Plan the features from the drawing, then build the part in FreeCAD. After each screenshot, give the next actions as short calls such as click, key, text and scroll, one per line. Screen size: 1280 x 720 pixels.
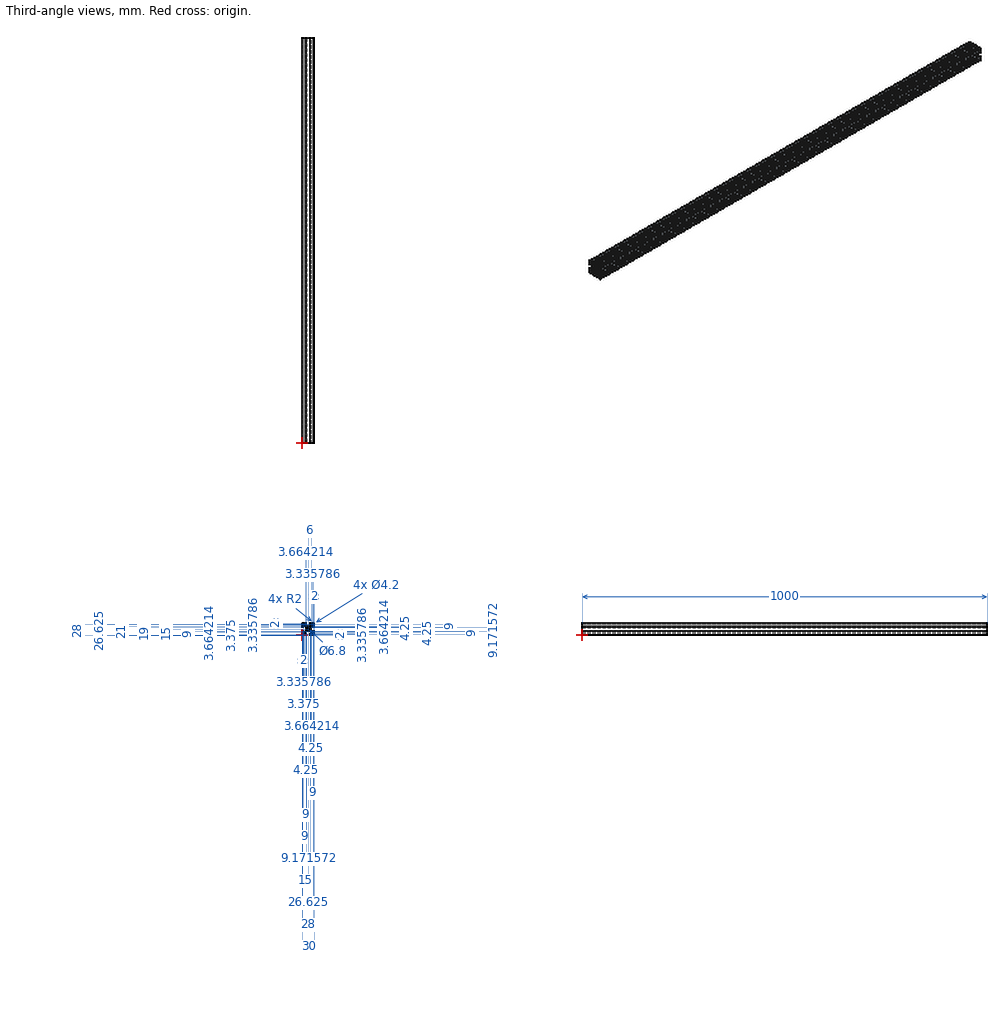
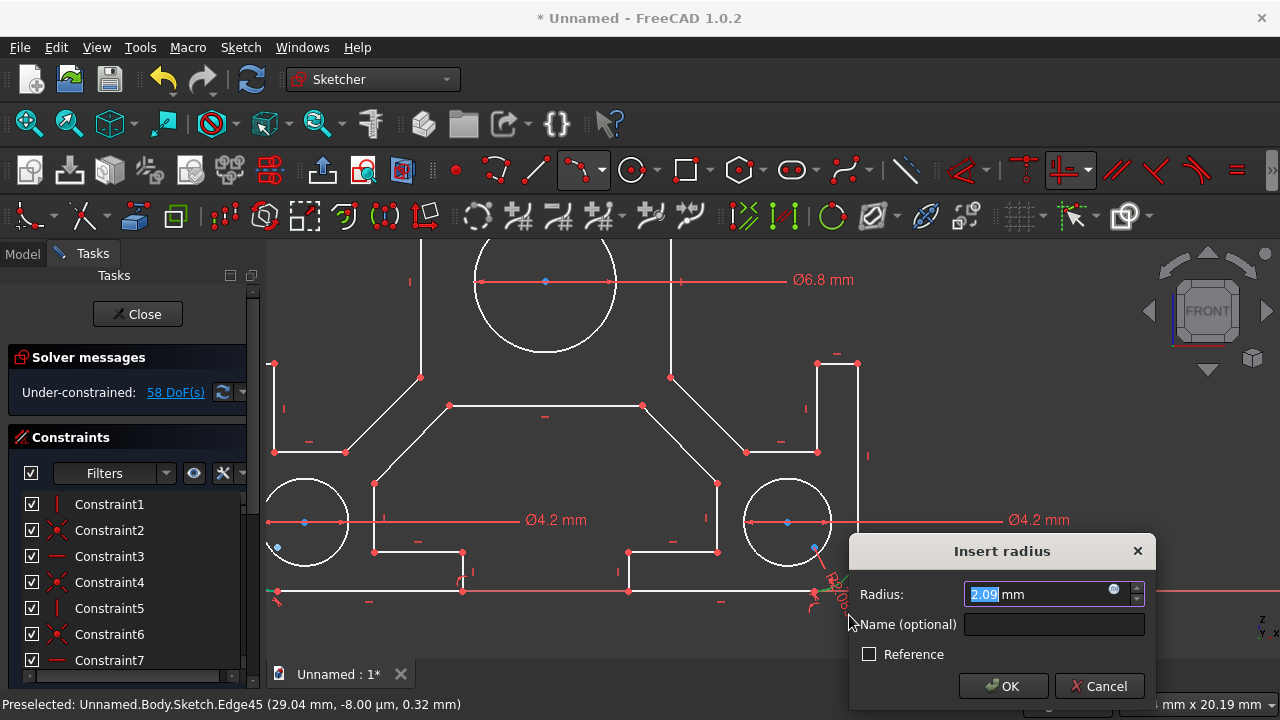
text(2)
key(Return)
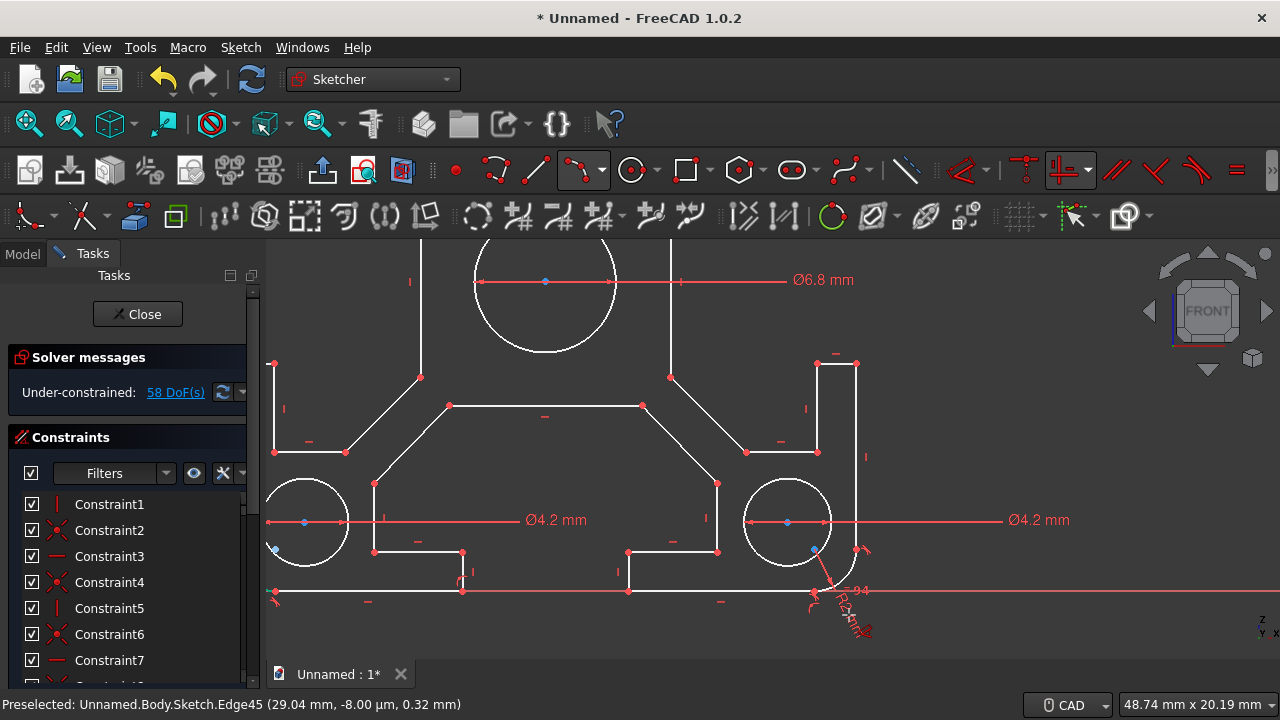
scroll(834, 588, down, 4)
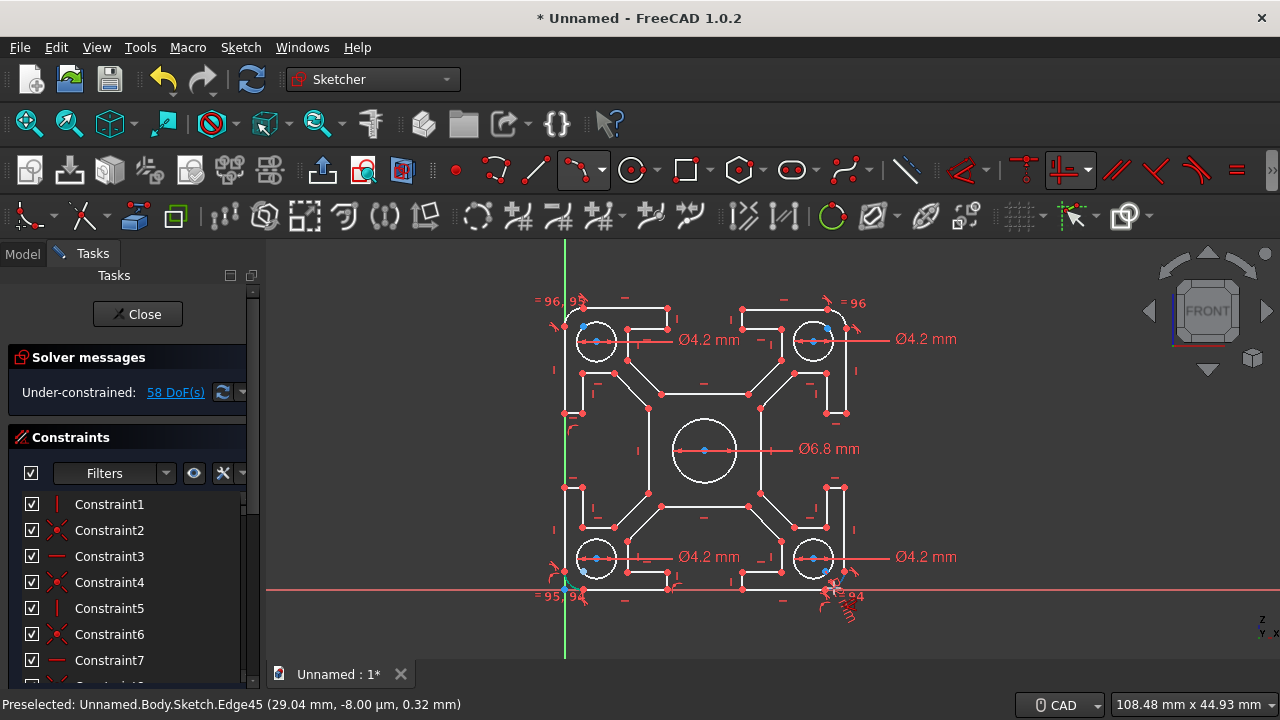
click(846, 354)
click(880, 371)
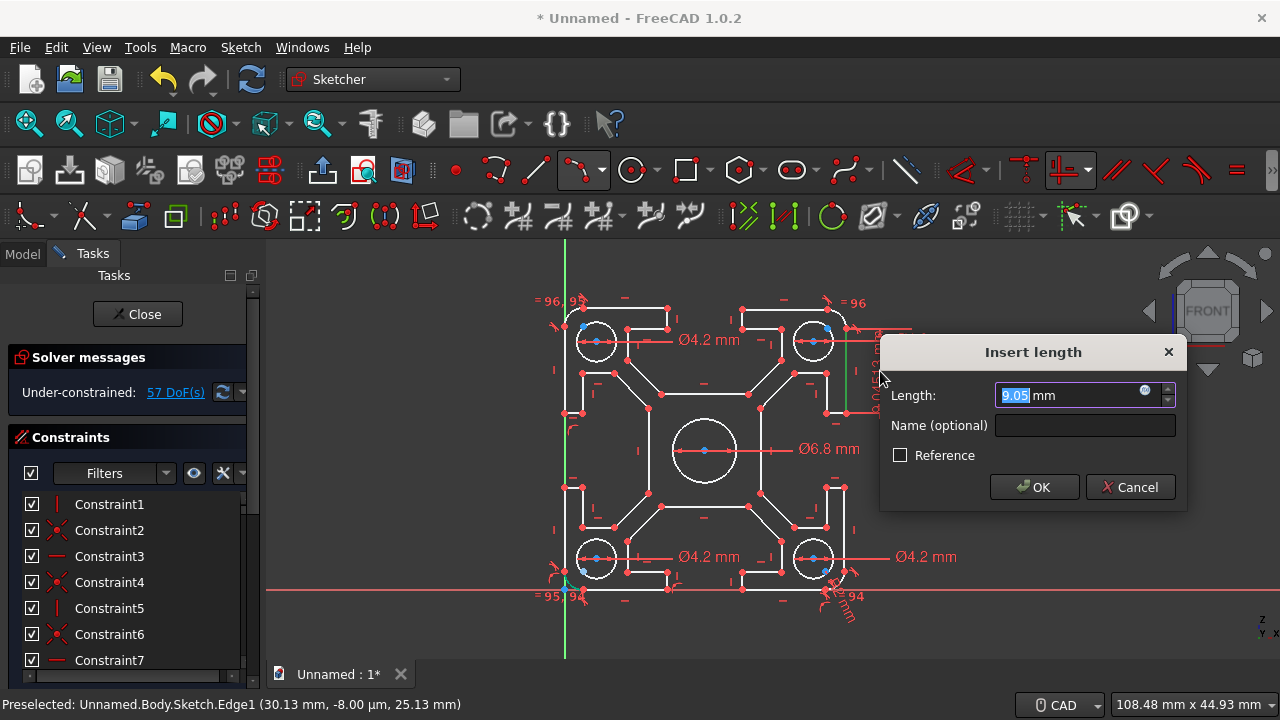
text(9)
key(Return)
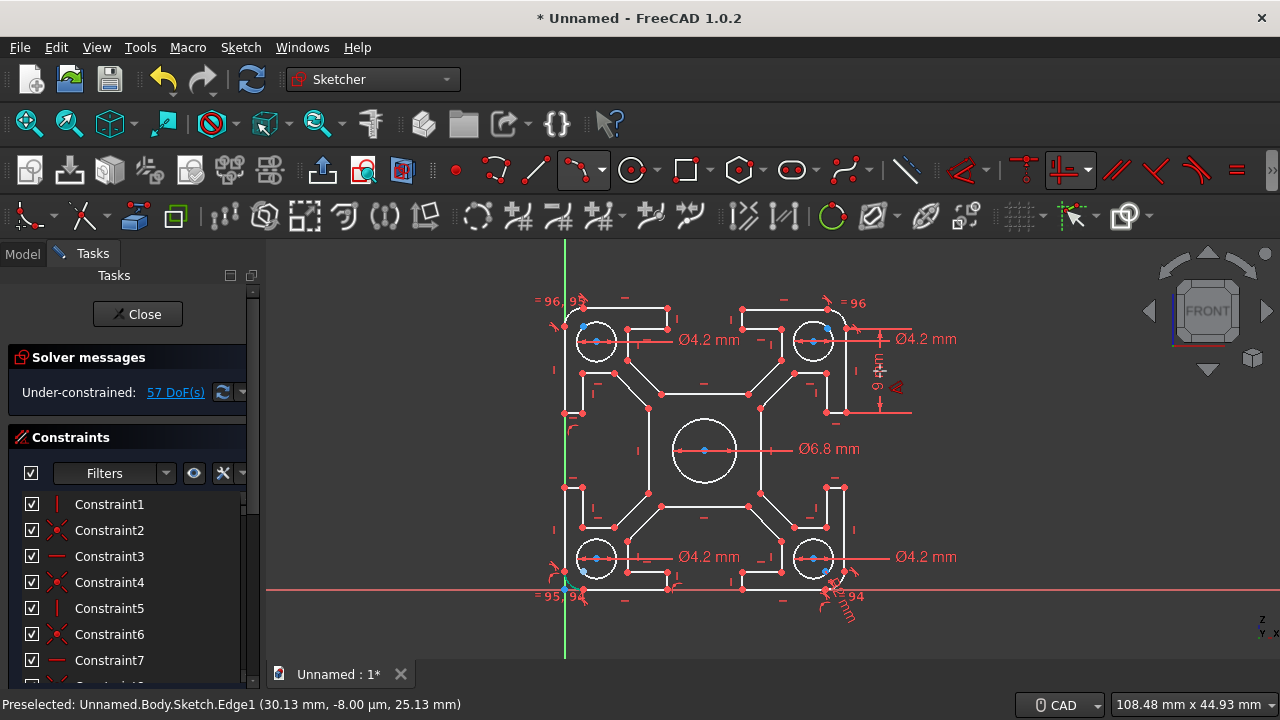
scroll(836, 413, up, 4)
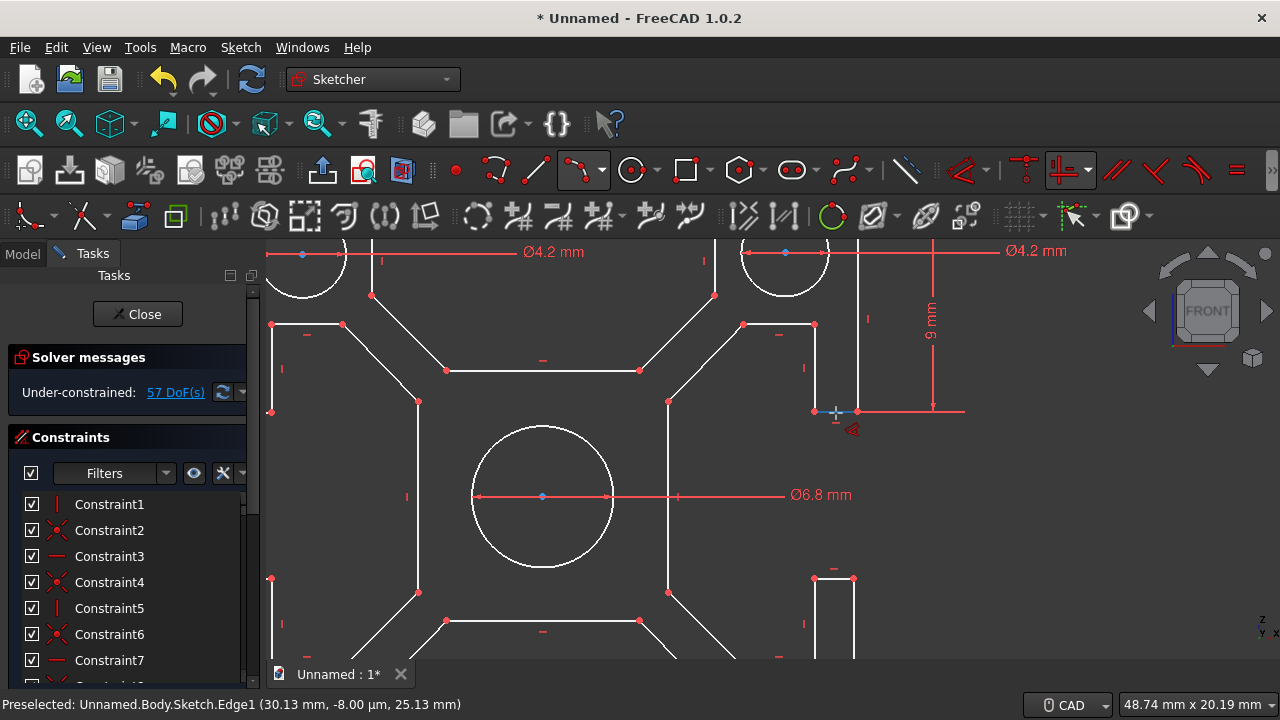
click(836, 412)
click(836, 378)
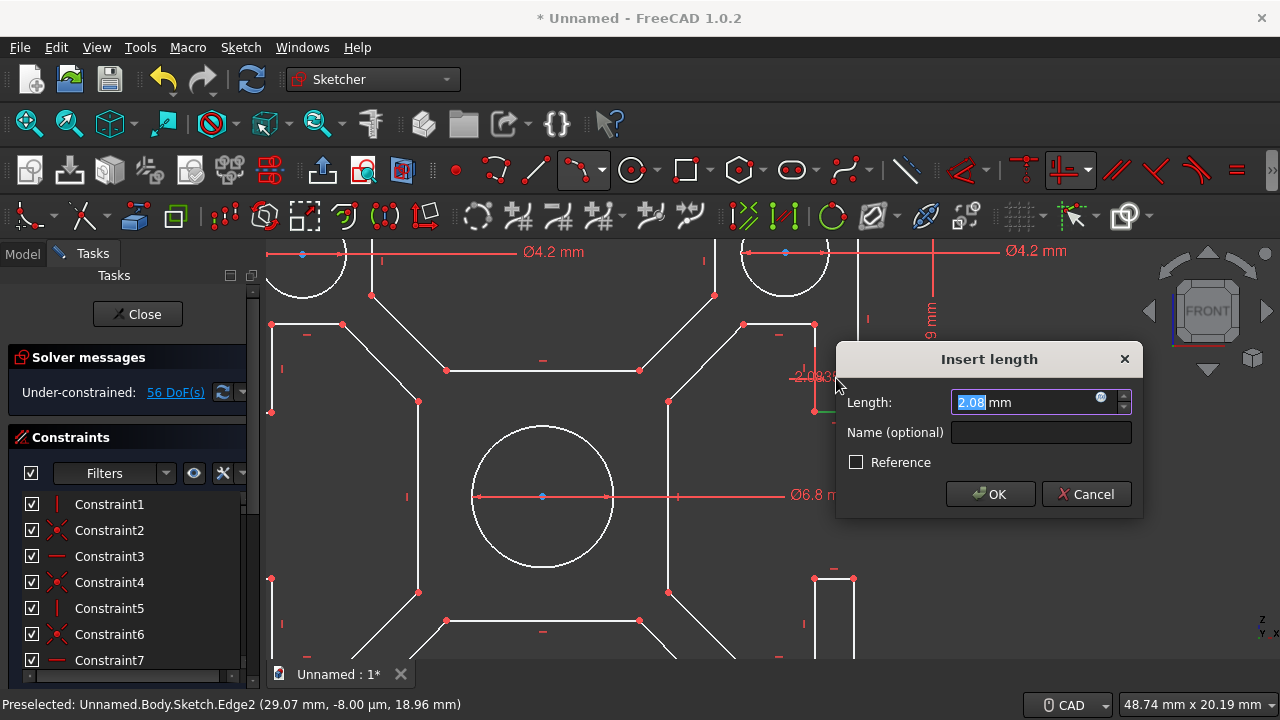
text(2)
key(Return)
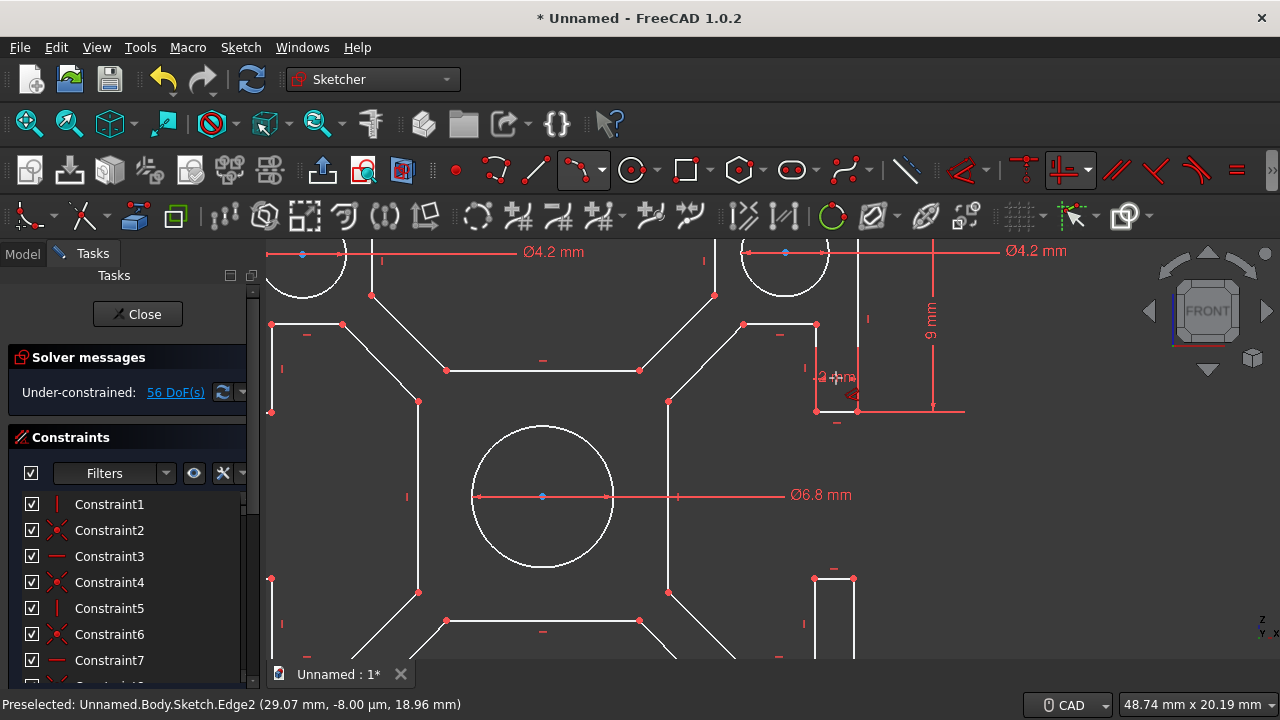
click(826, 579)
click(834, 613)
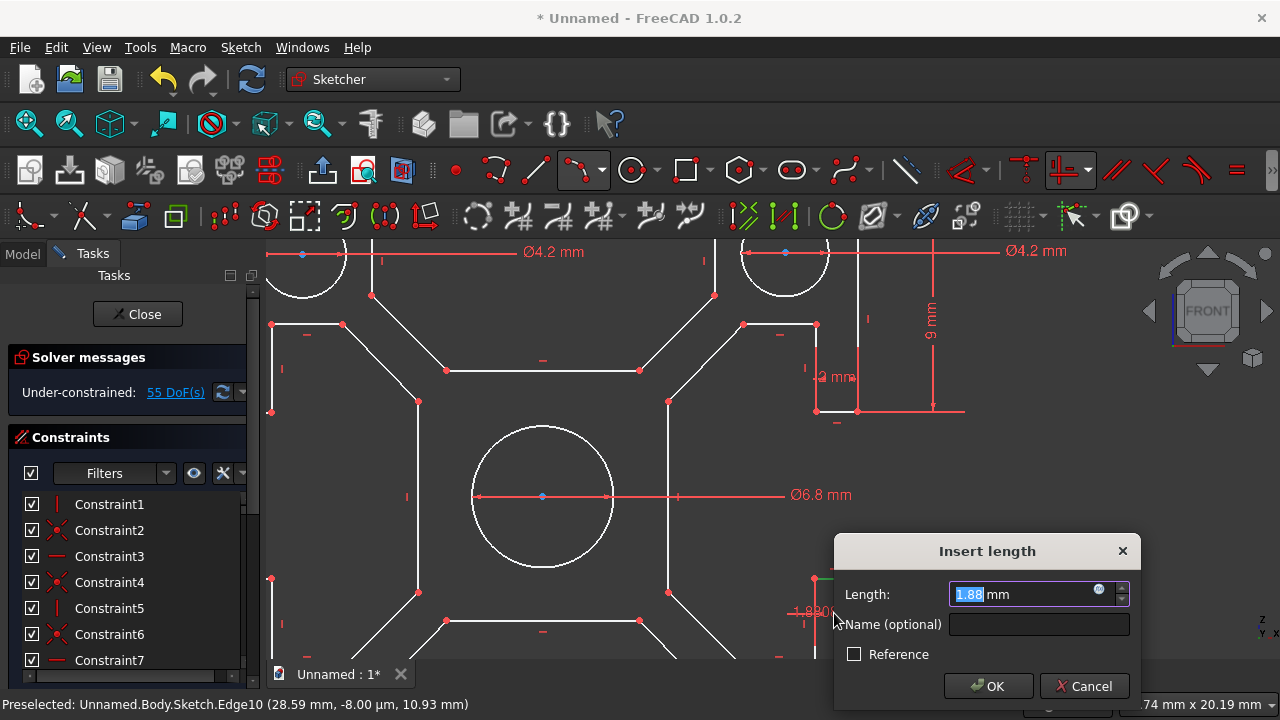
text(2)
key(Return)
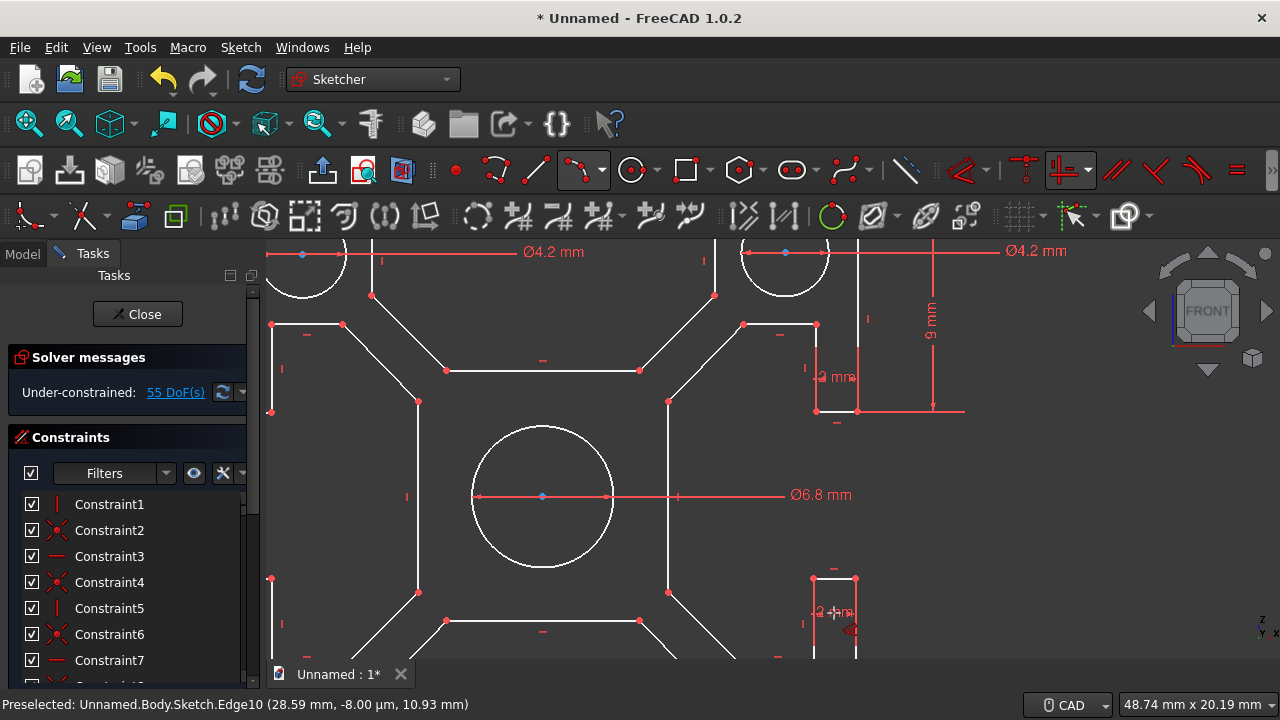
click(856, 616)
click(890, 587)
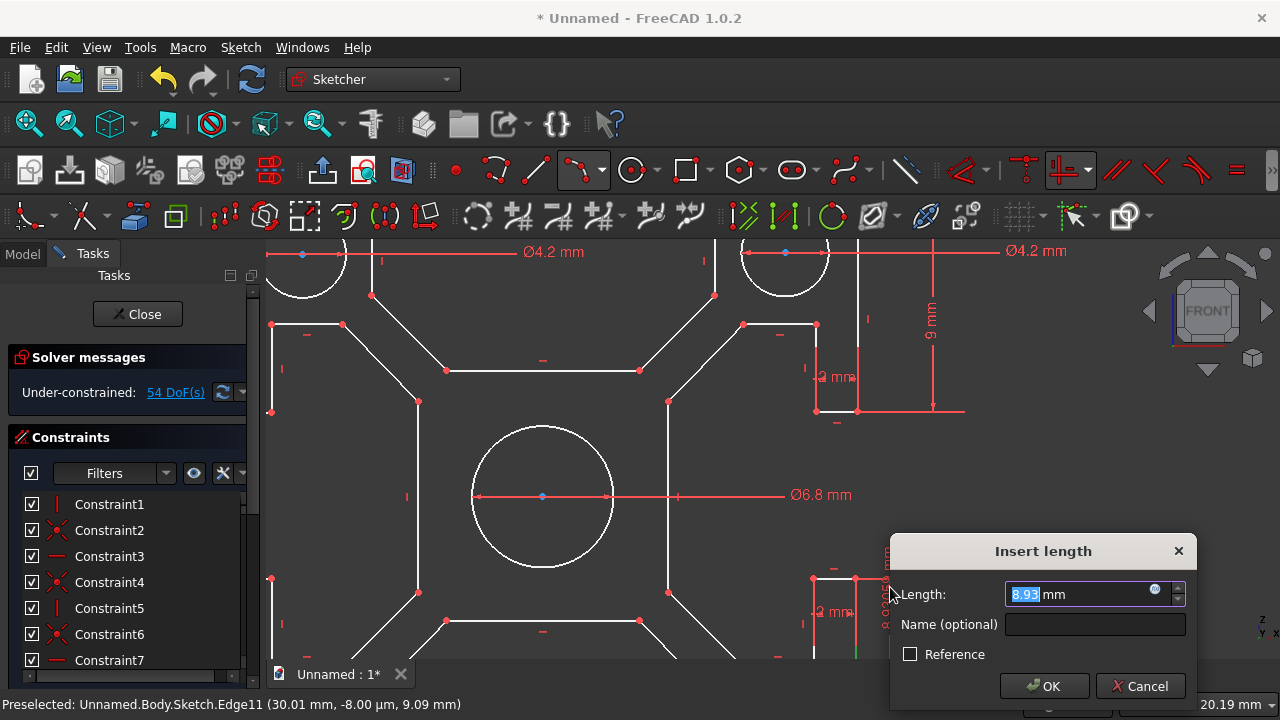
text(9)
key(Return)